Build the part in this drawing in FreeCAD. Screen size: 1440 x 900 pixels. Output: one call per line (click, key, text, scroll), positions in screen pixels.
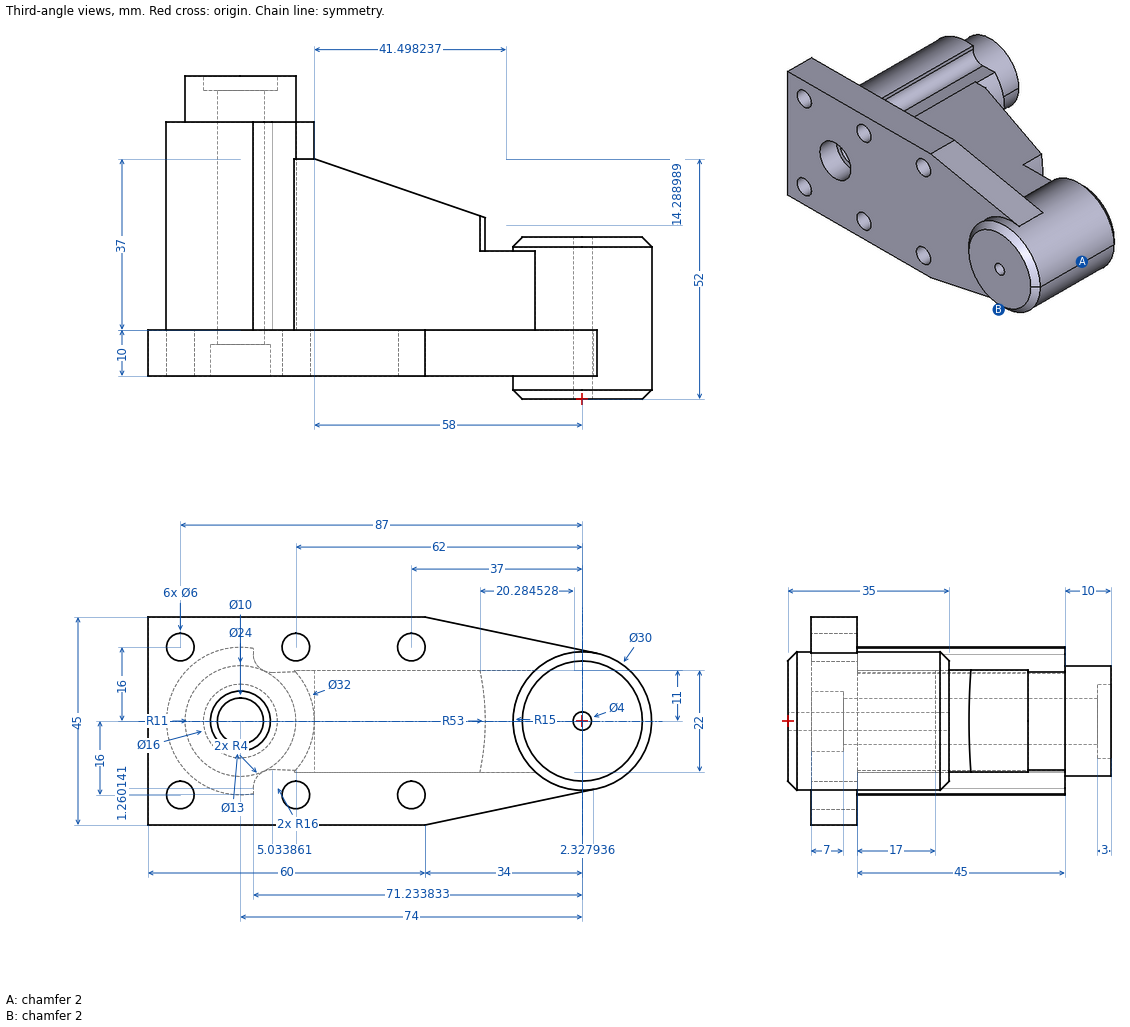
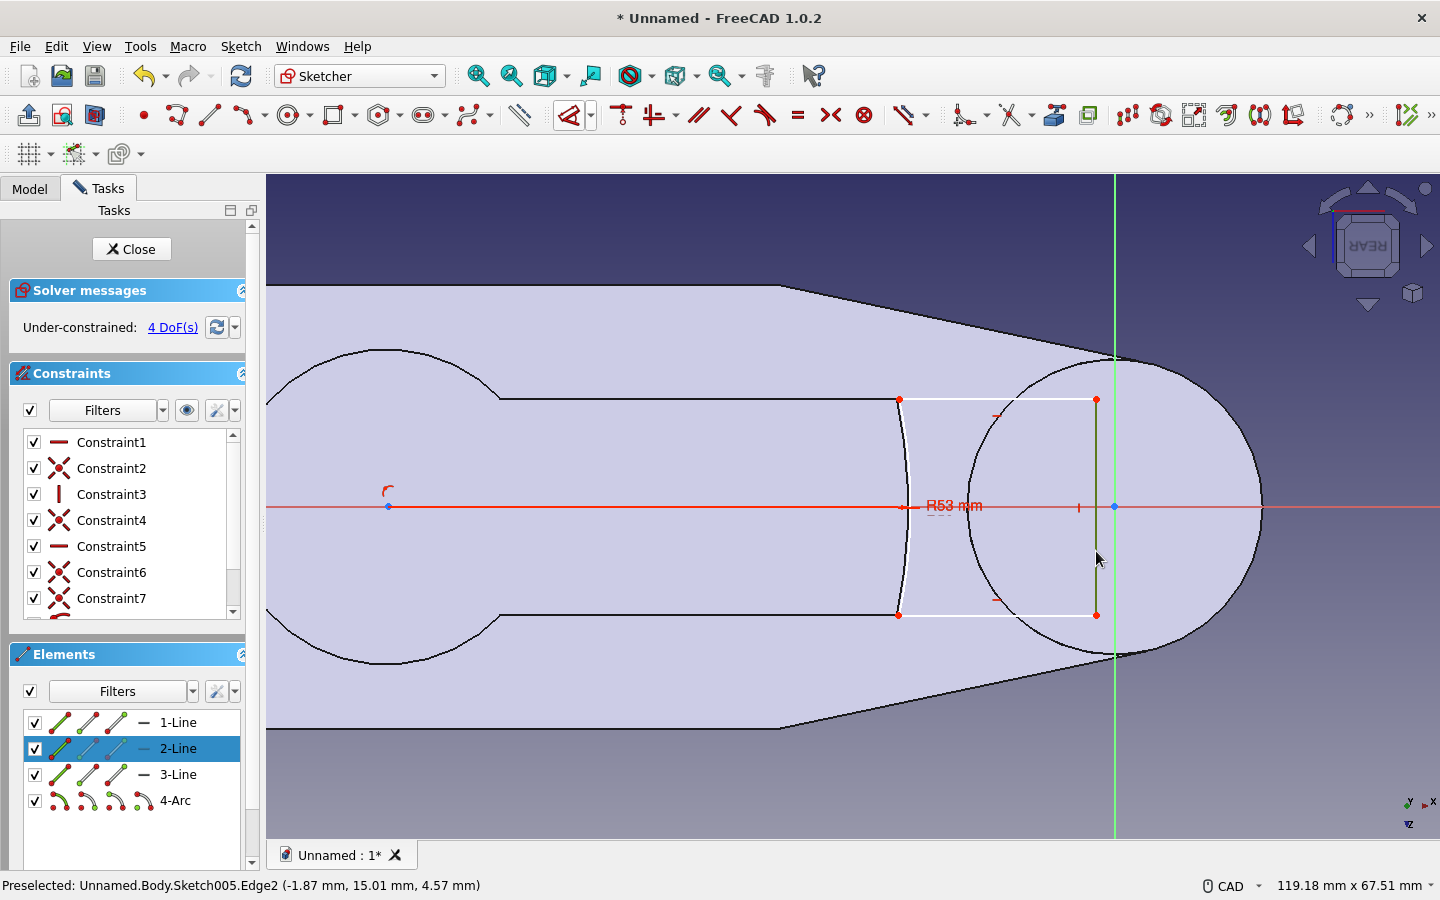
click(590, 116)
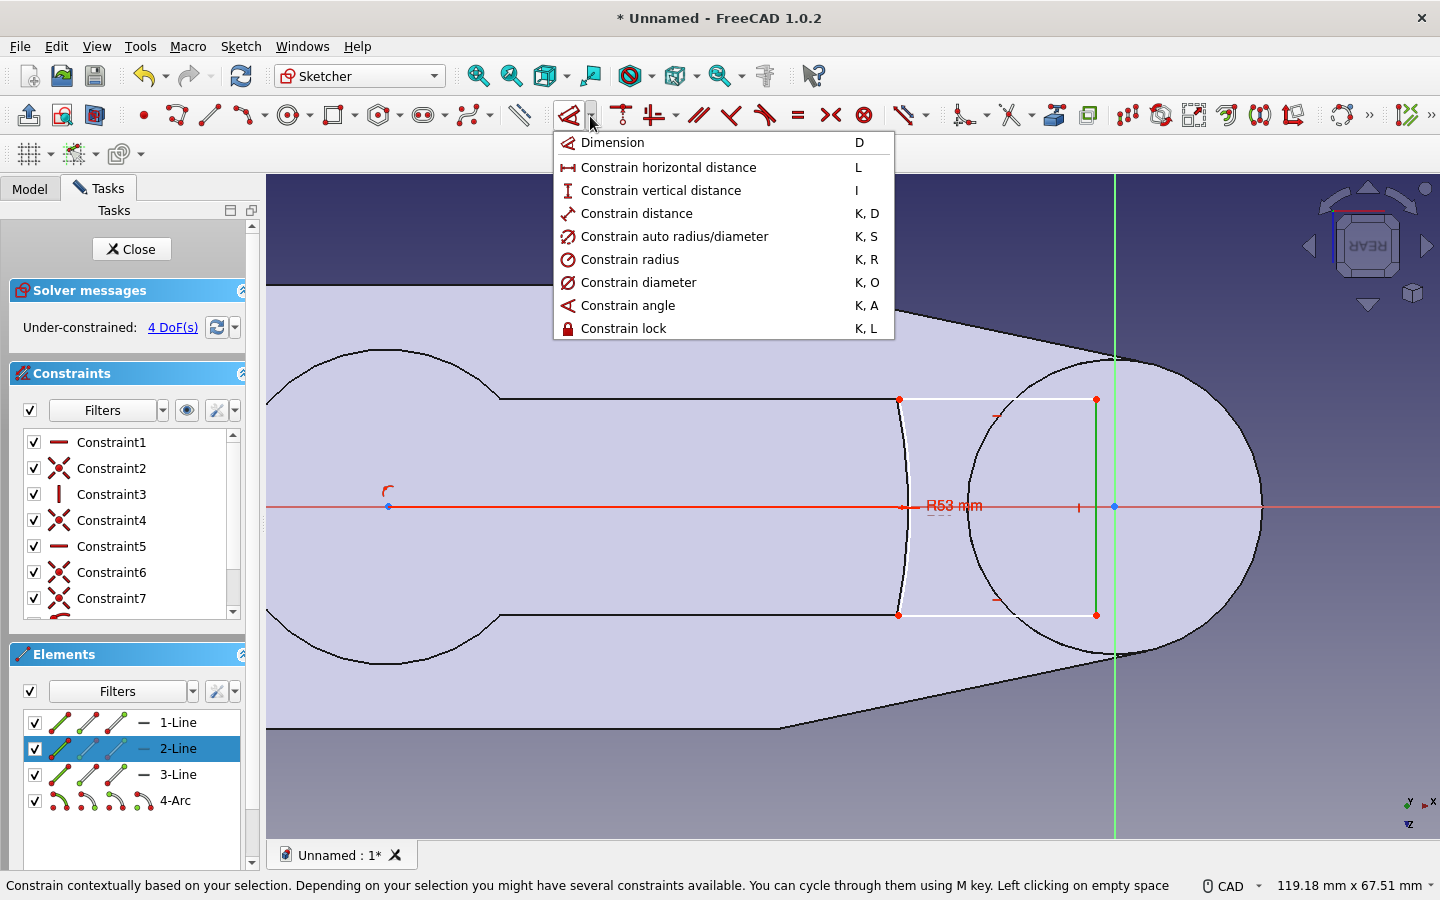
click(724, 190)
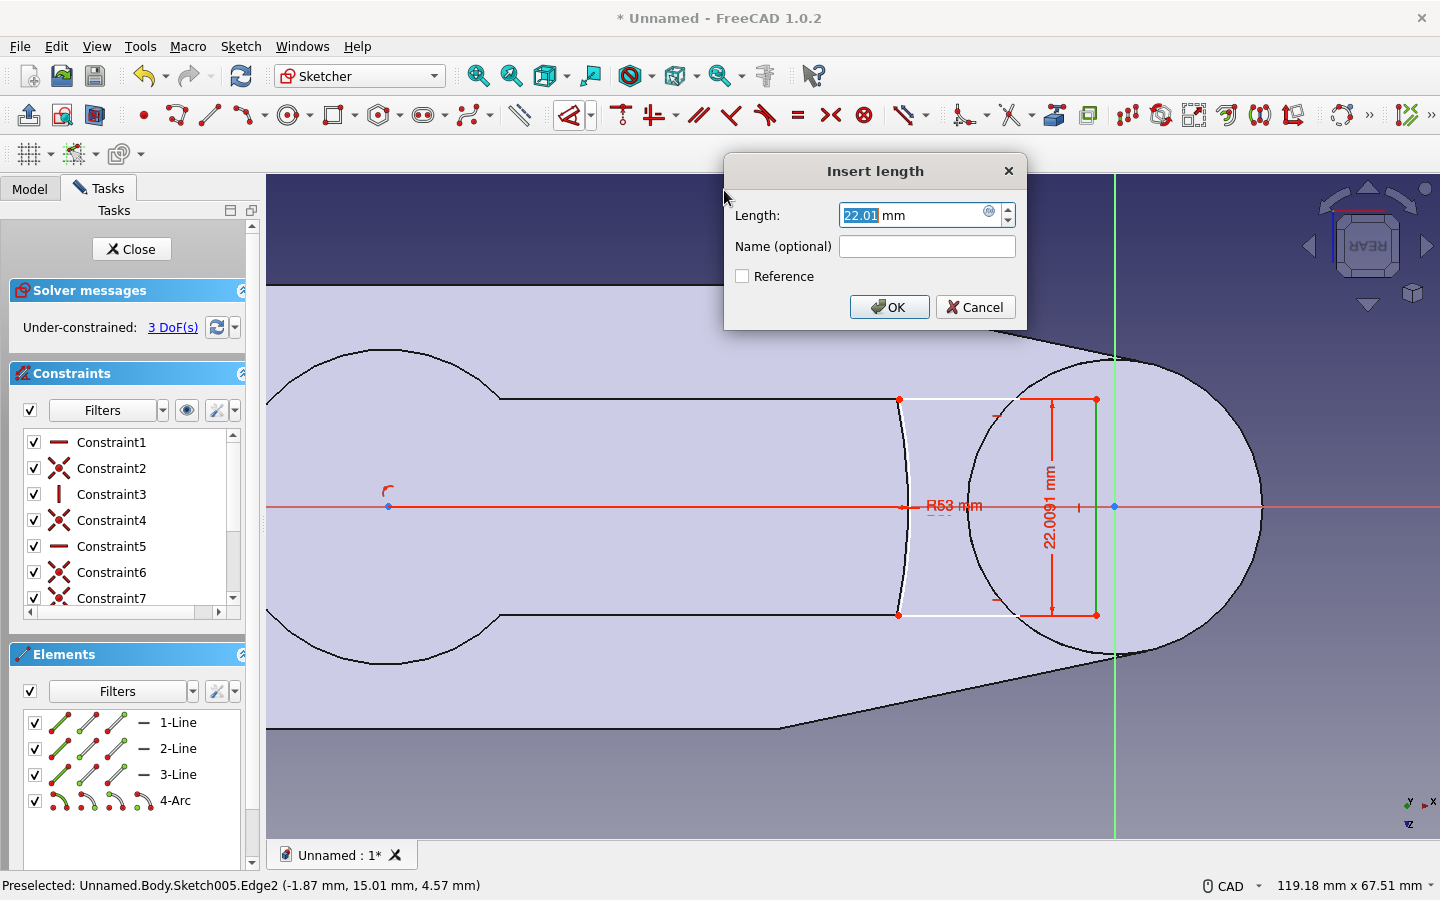
text(22)
key(Return)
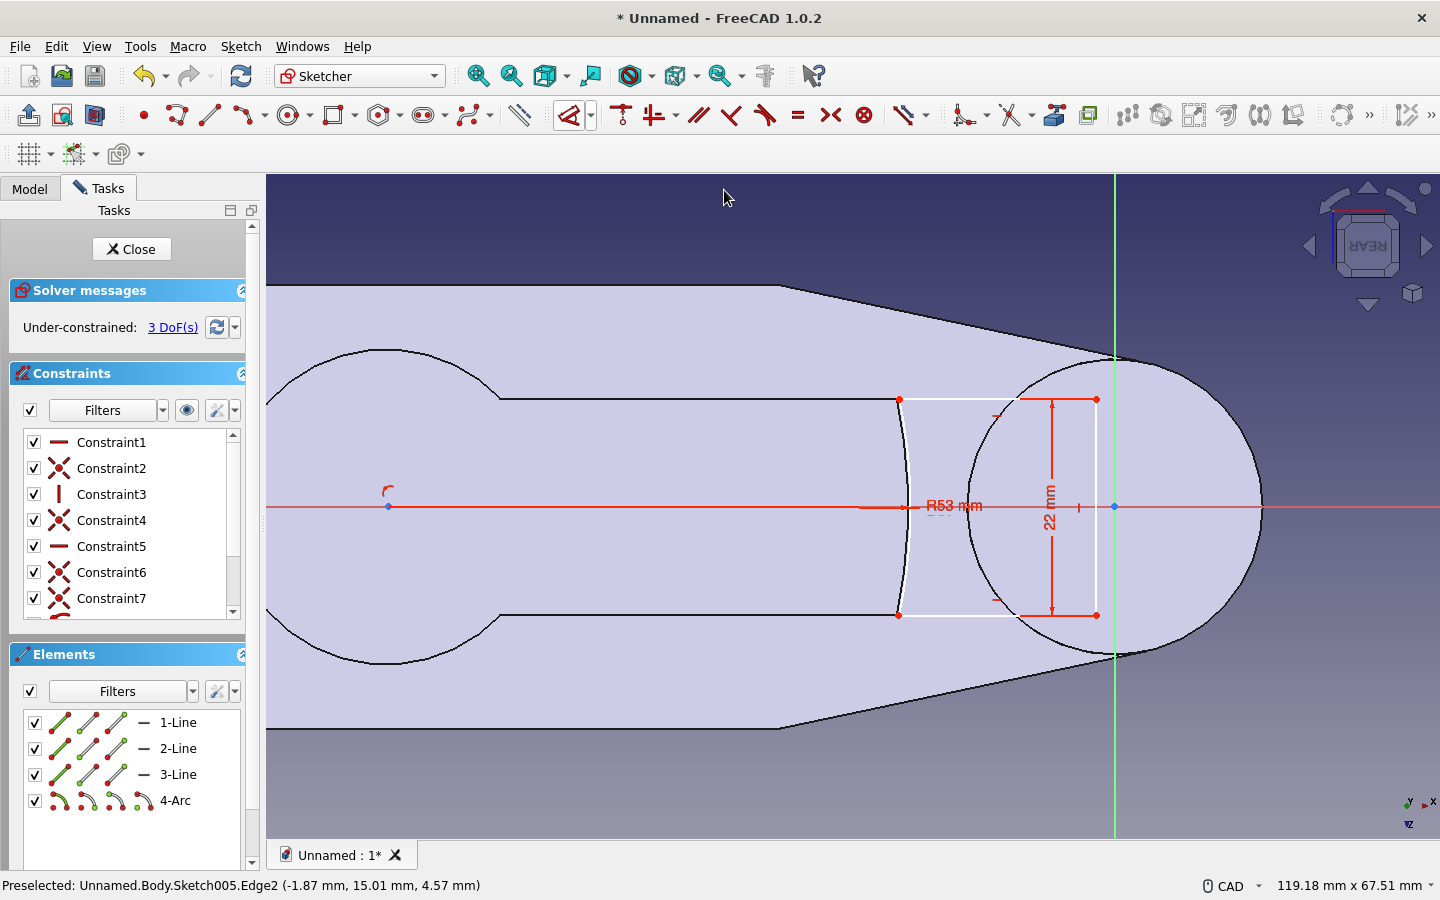
click(899, 616)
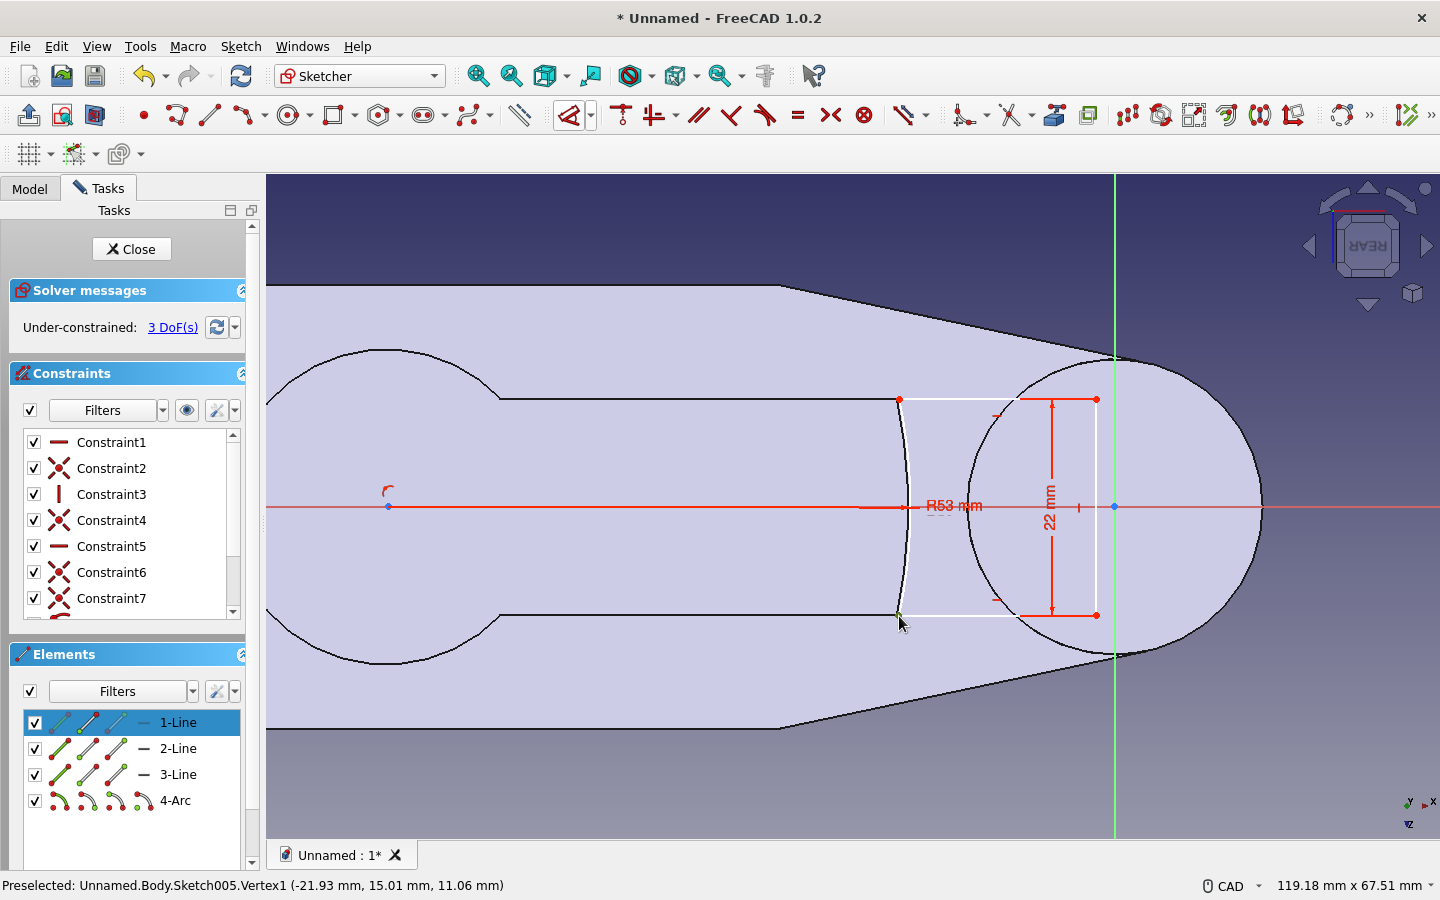
key(i)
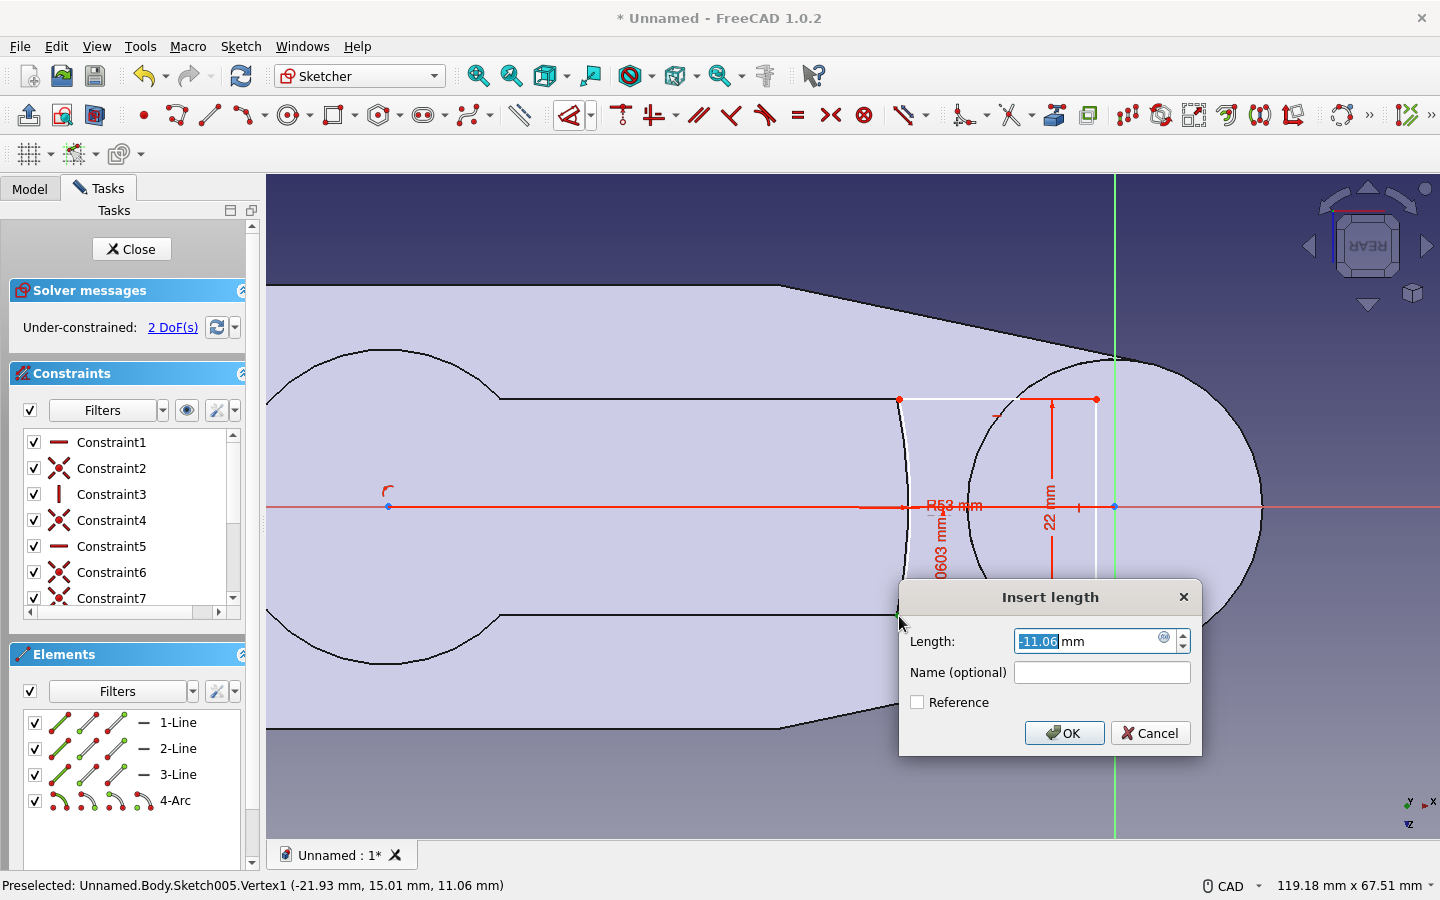
text(-11)
key(Return)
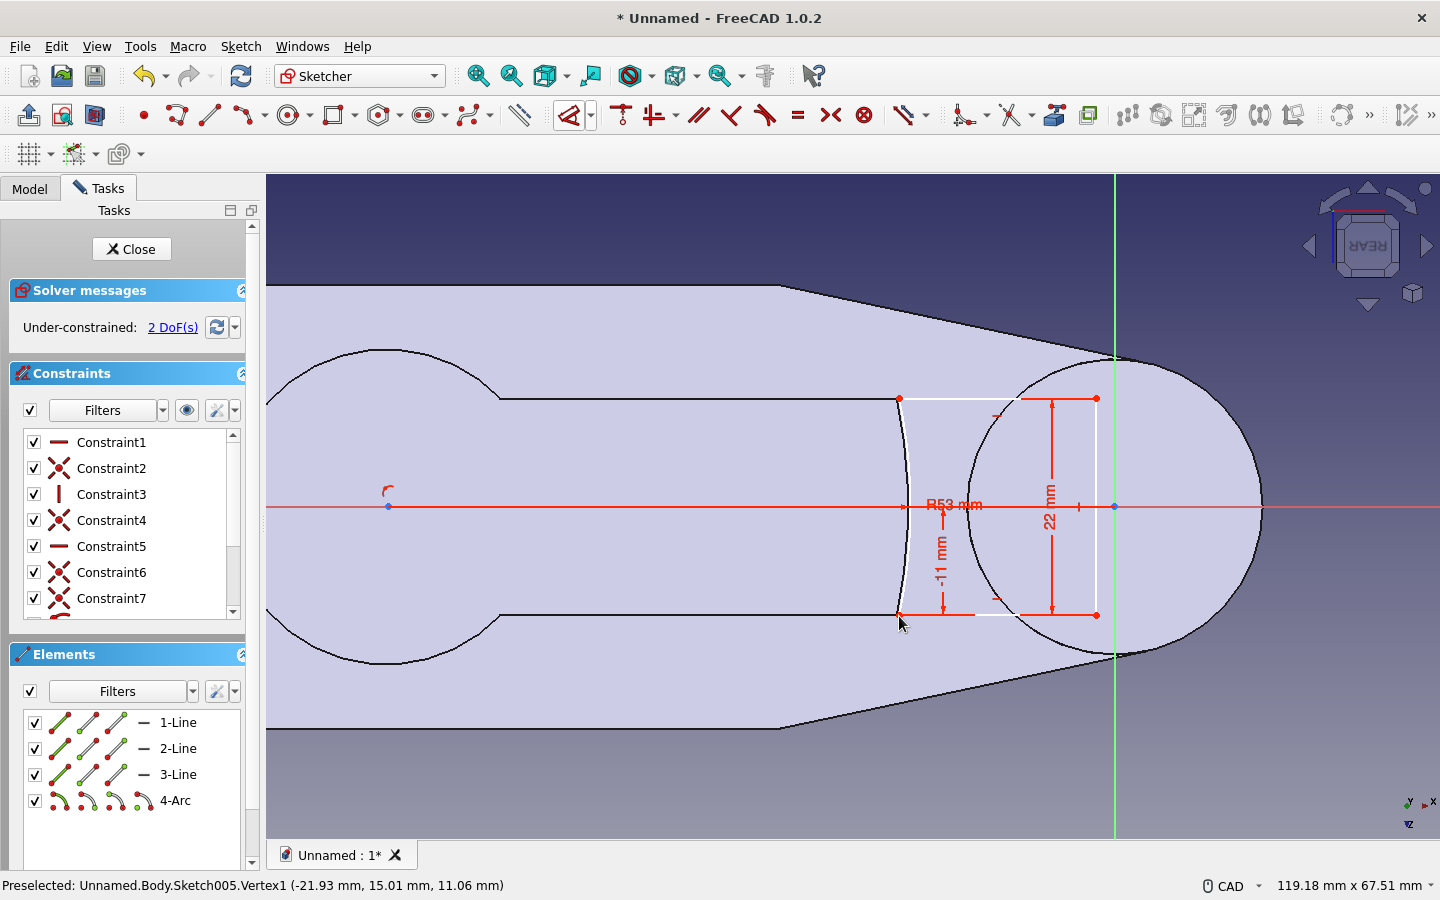
click(388, 507)